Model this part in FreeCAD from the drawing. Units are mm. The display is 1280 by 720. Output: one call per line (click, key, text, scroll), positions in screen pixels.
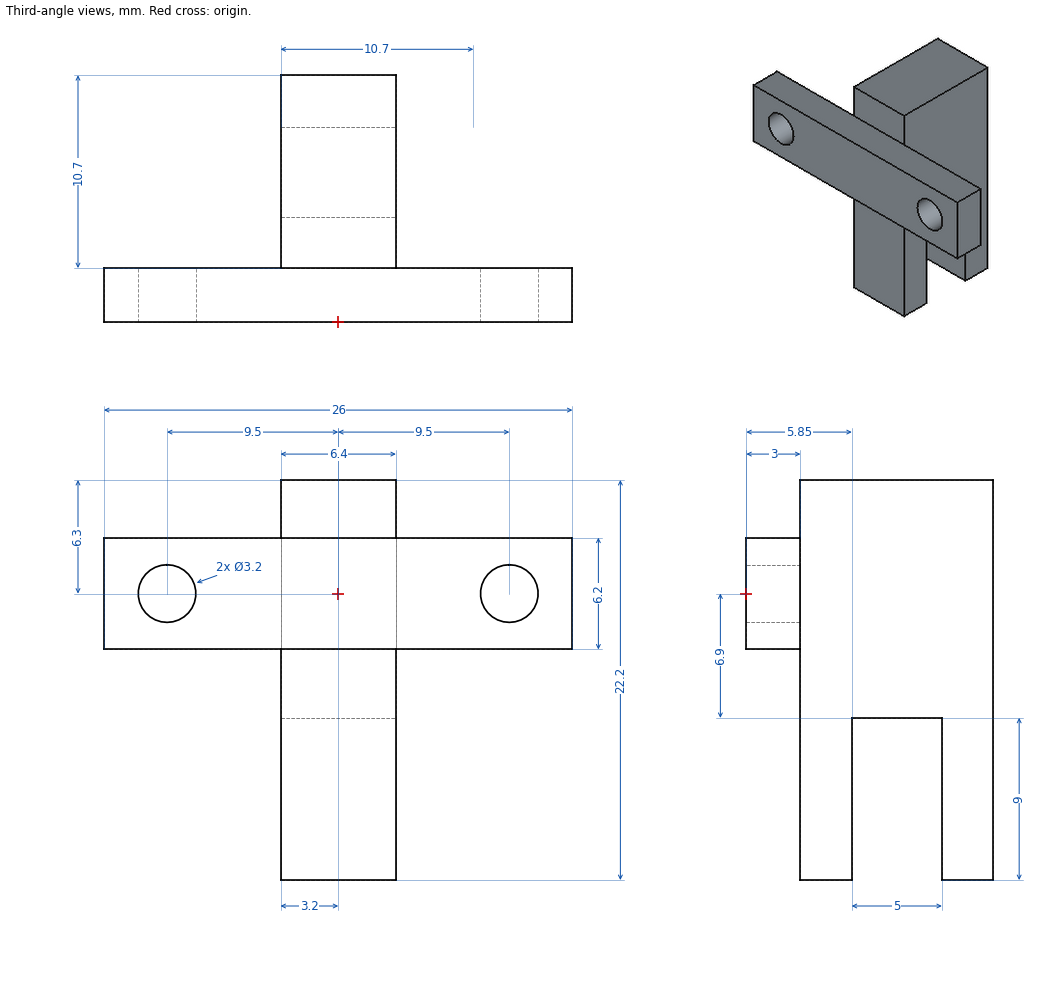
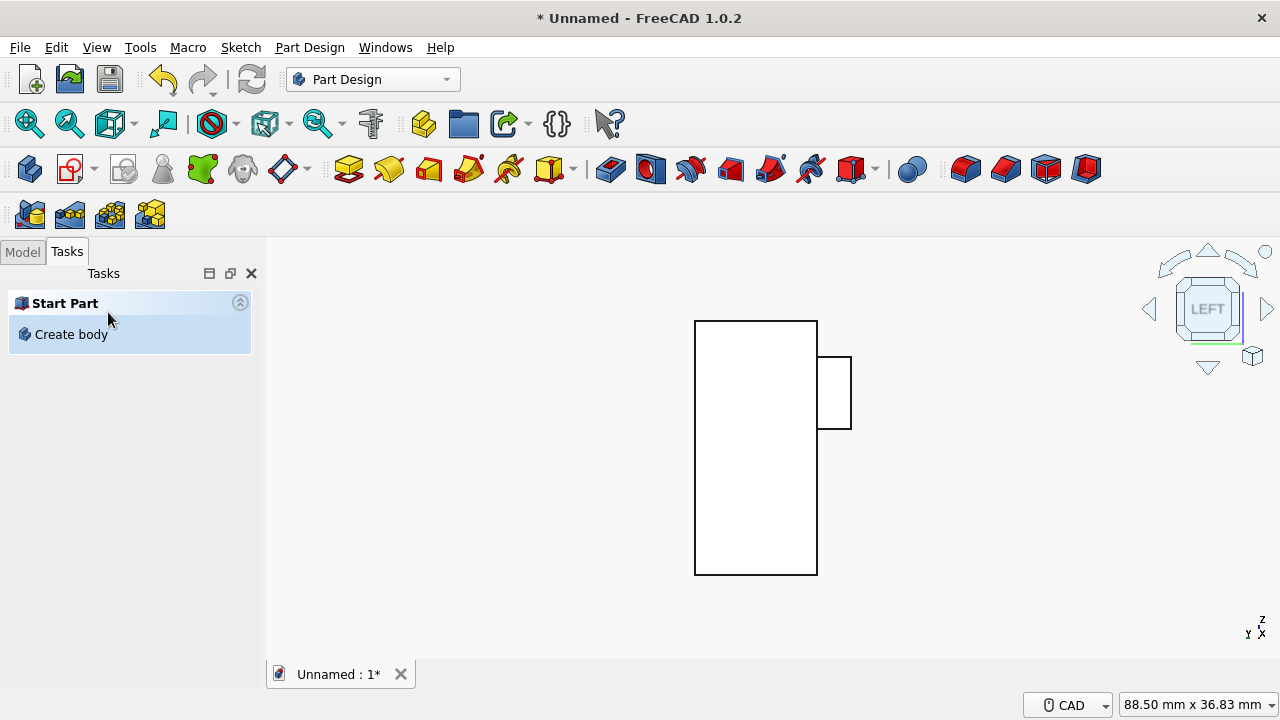
click(756, 447)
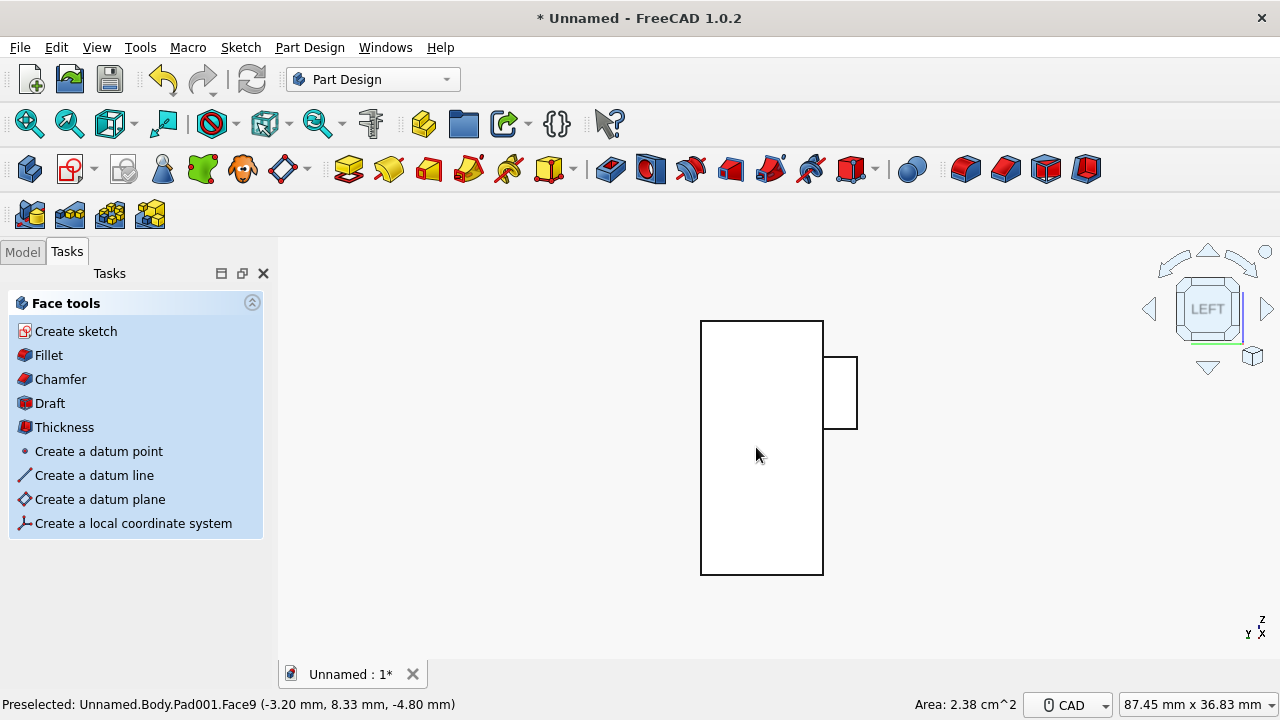
click(70, 170)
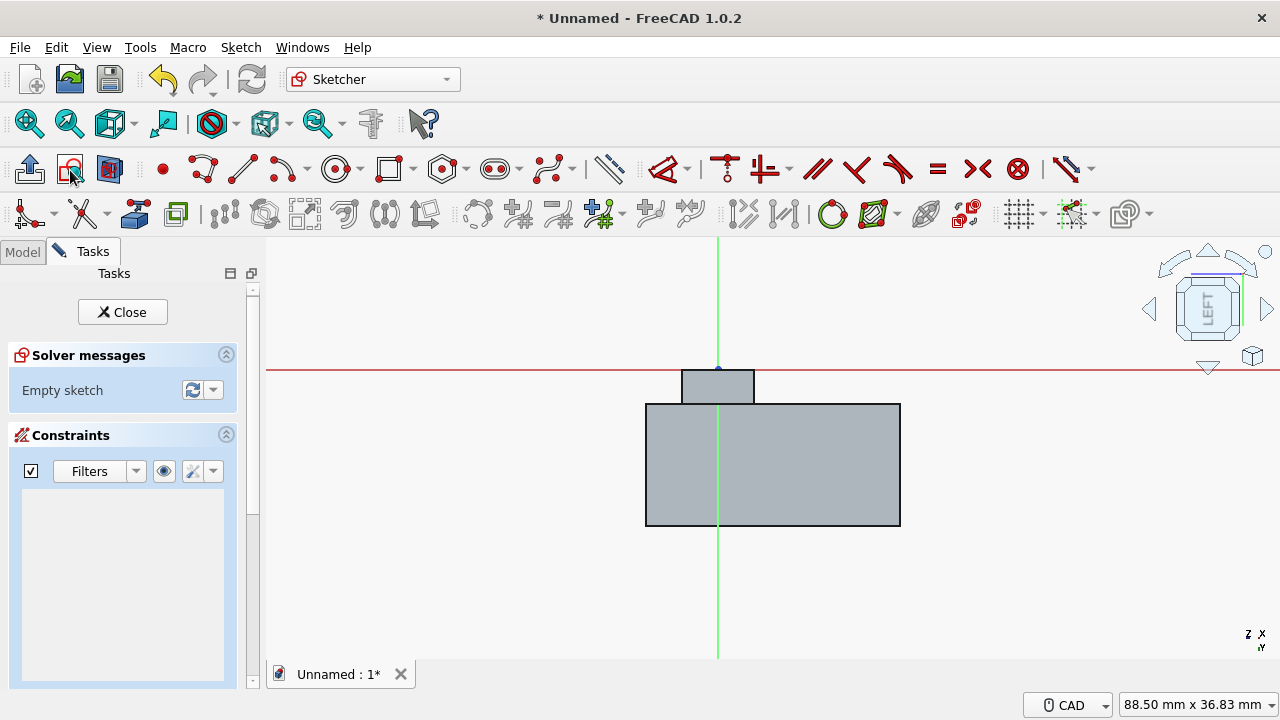
key(q)
key(s)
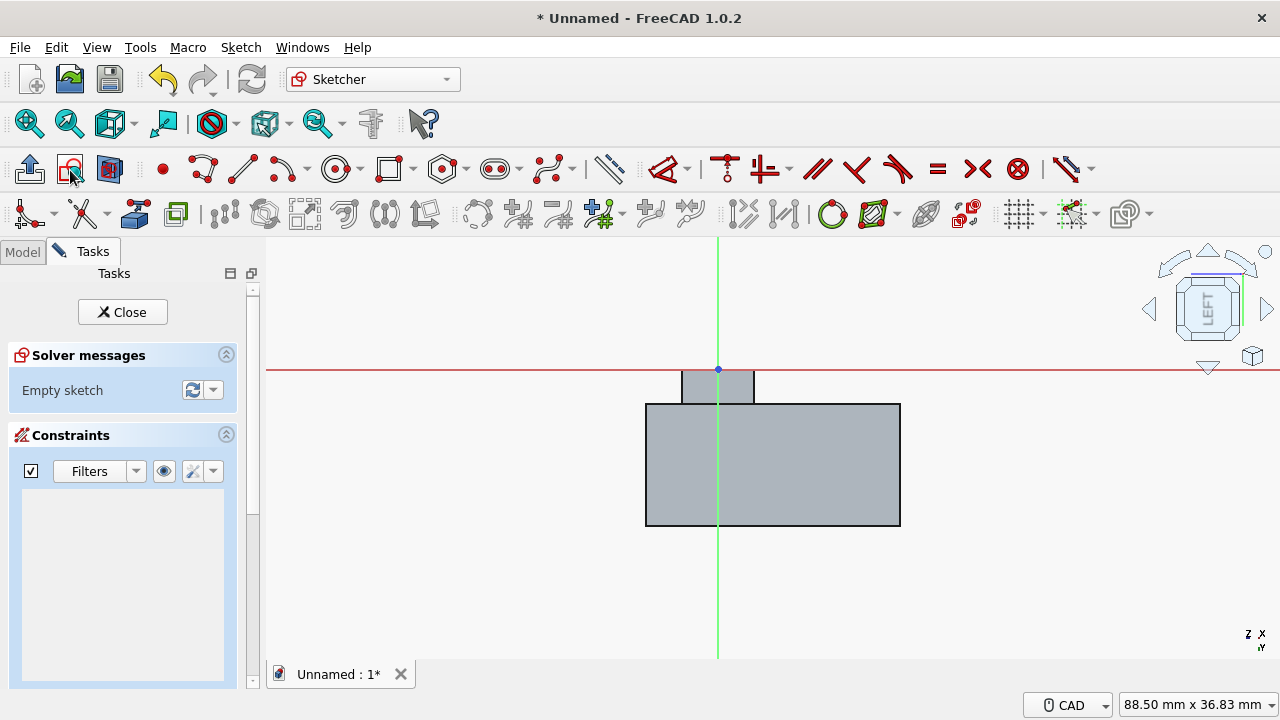
scroll(894, 418, up, 4)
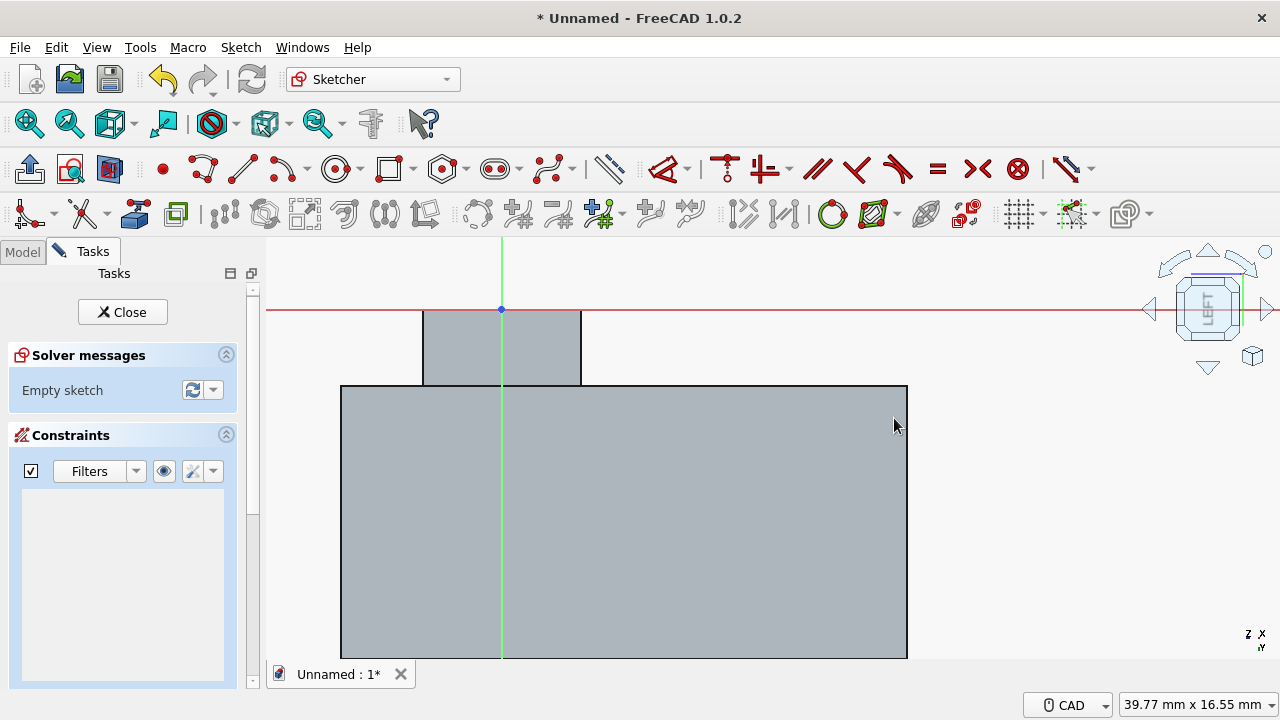
key(g)
key(r)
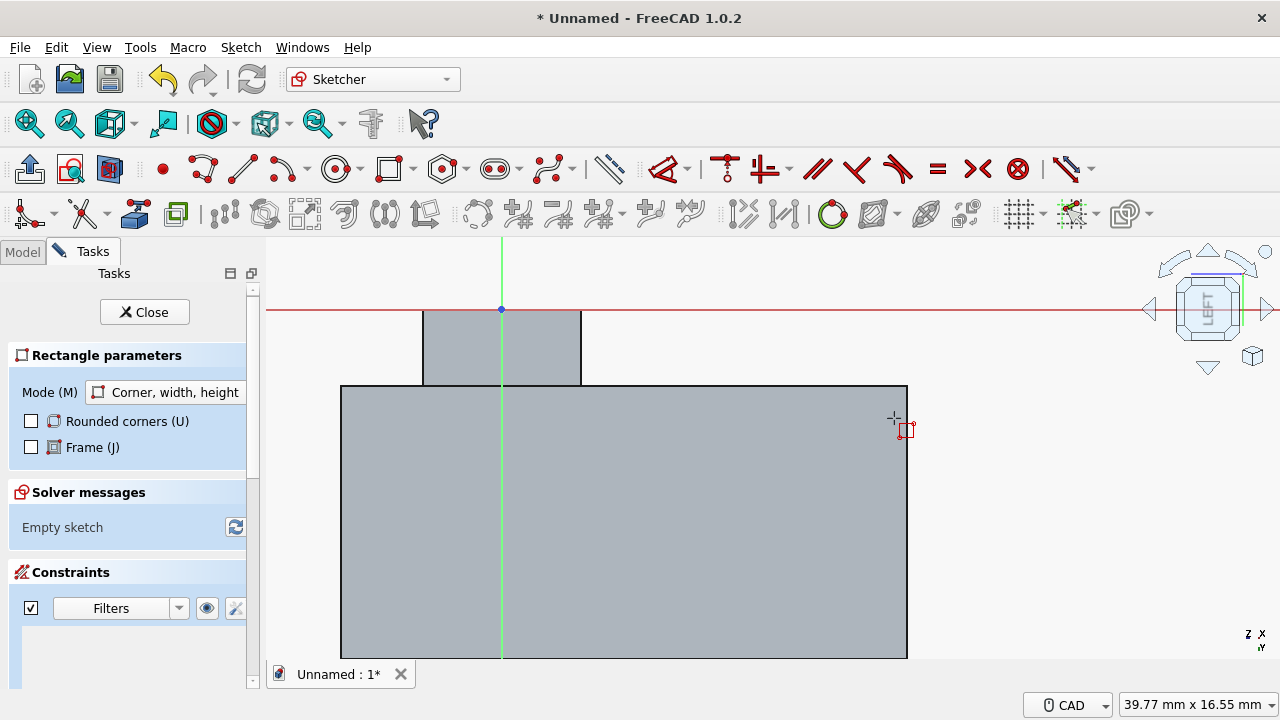
click(677, 459)
move(907, 586)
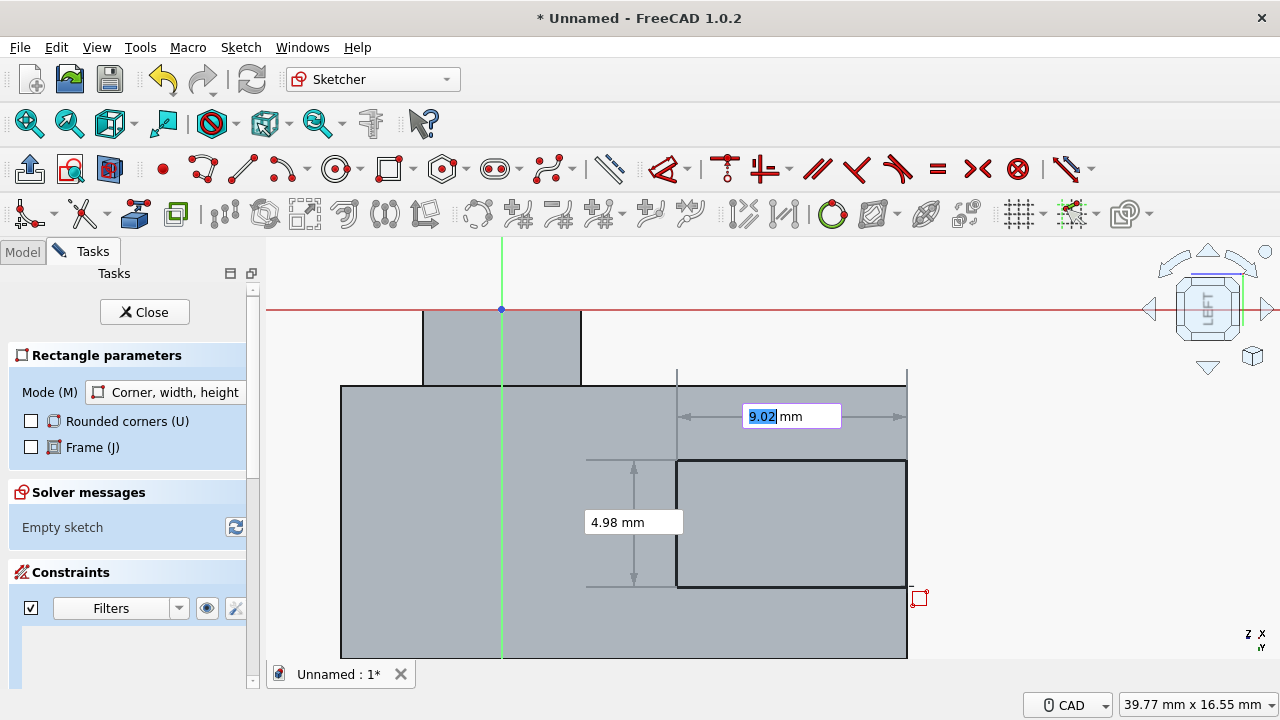
text(9)
key(Tab)
text(5)
key(Return)
key(Escape)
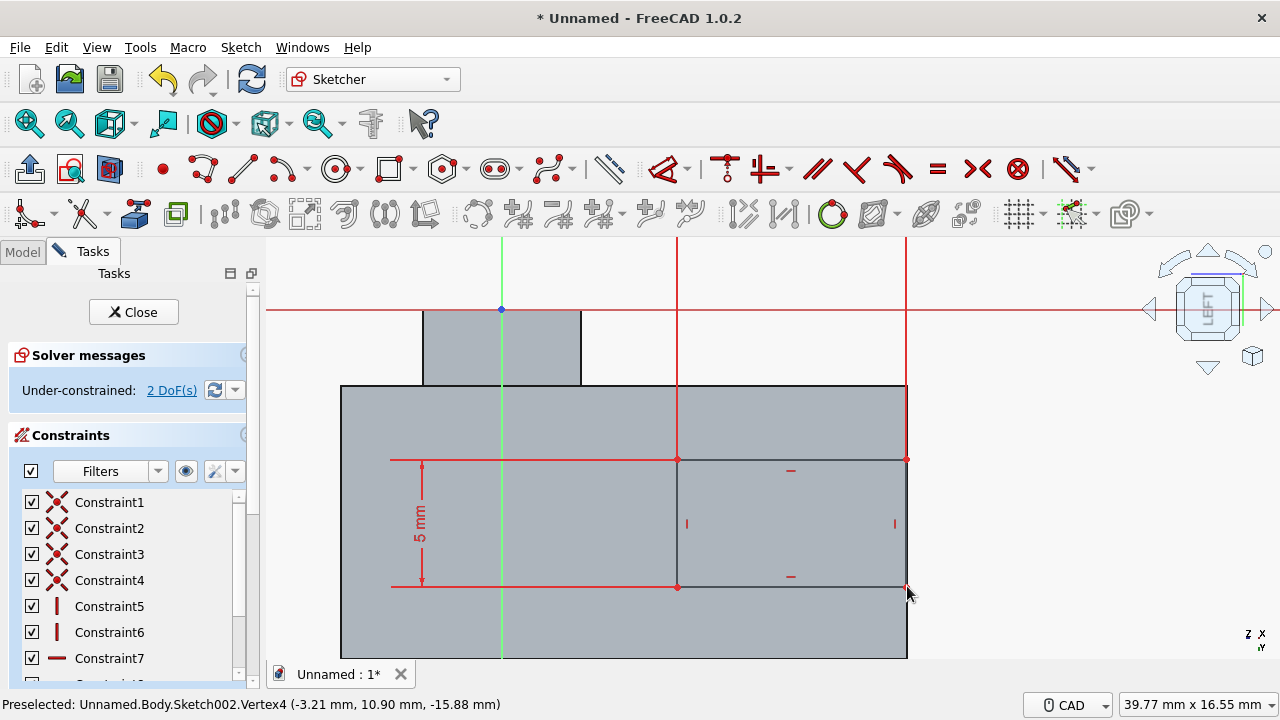
click(664, 170)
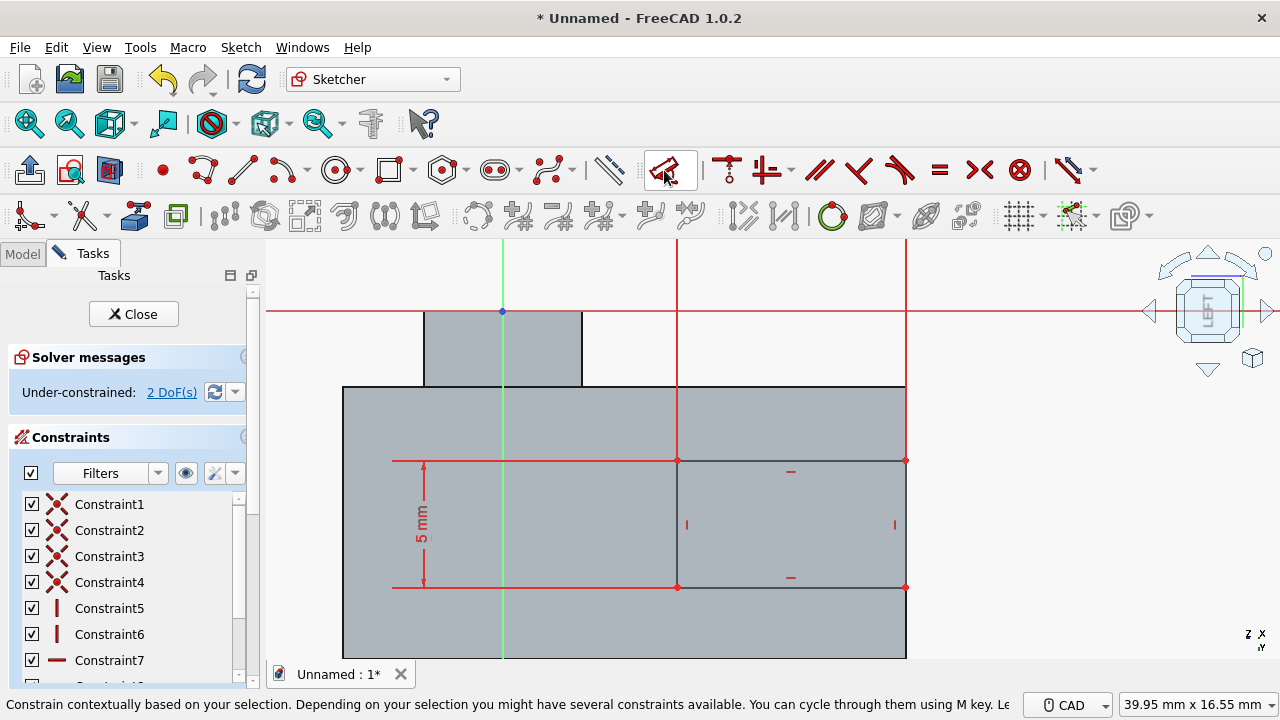
click(677, 461)
click(590, 277)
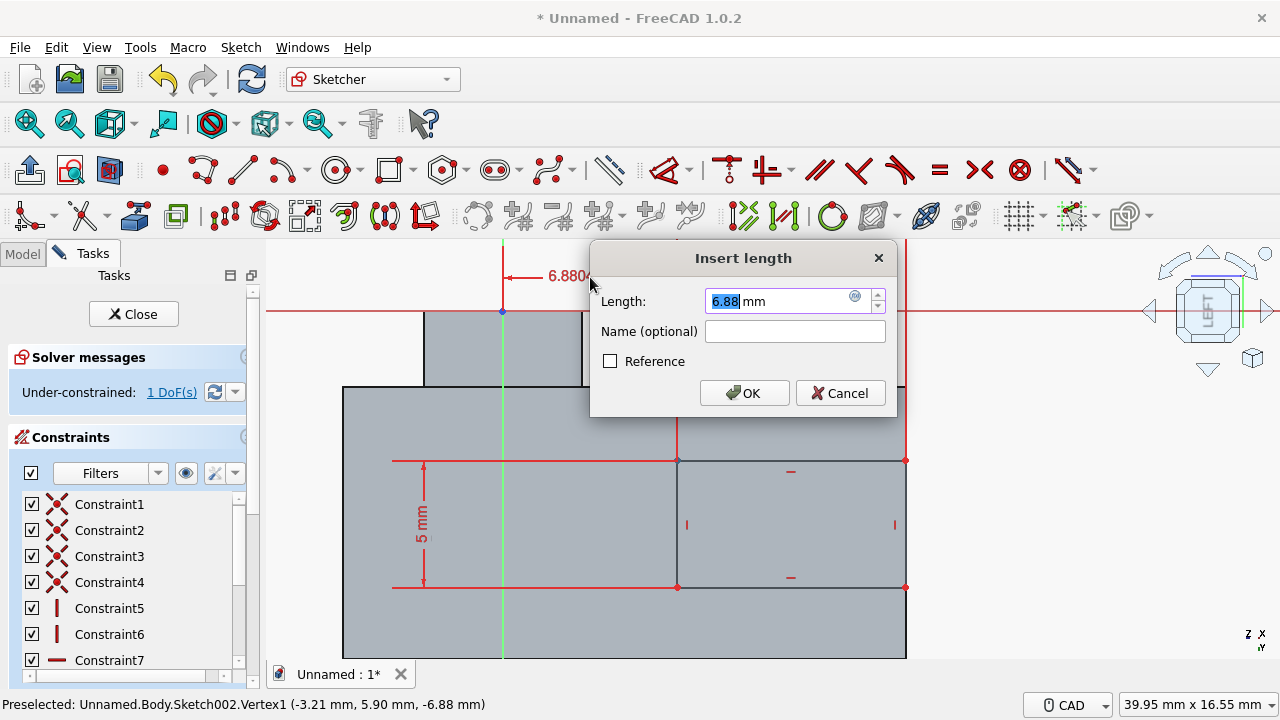
text(6.9)
key(Return)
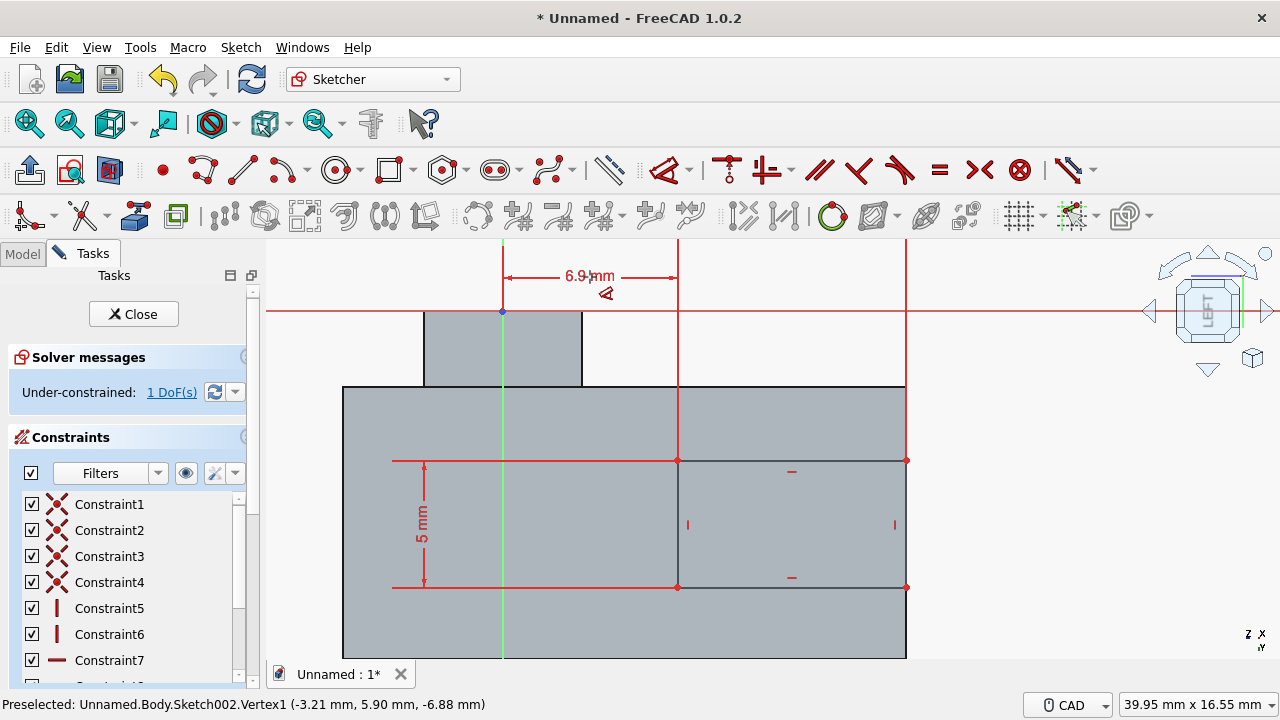
click(678, 461)
click(469, 386)